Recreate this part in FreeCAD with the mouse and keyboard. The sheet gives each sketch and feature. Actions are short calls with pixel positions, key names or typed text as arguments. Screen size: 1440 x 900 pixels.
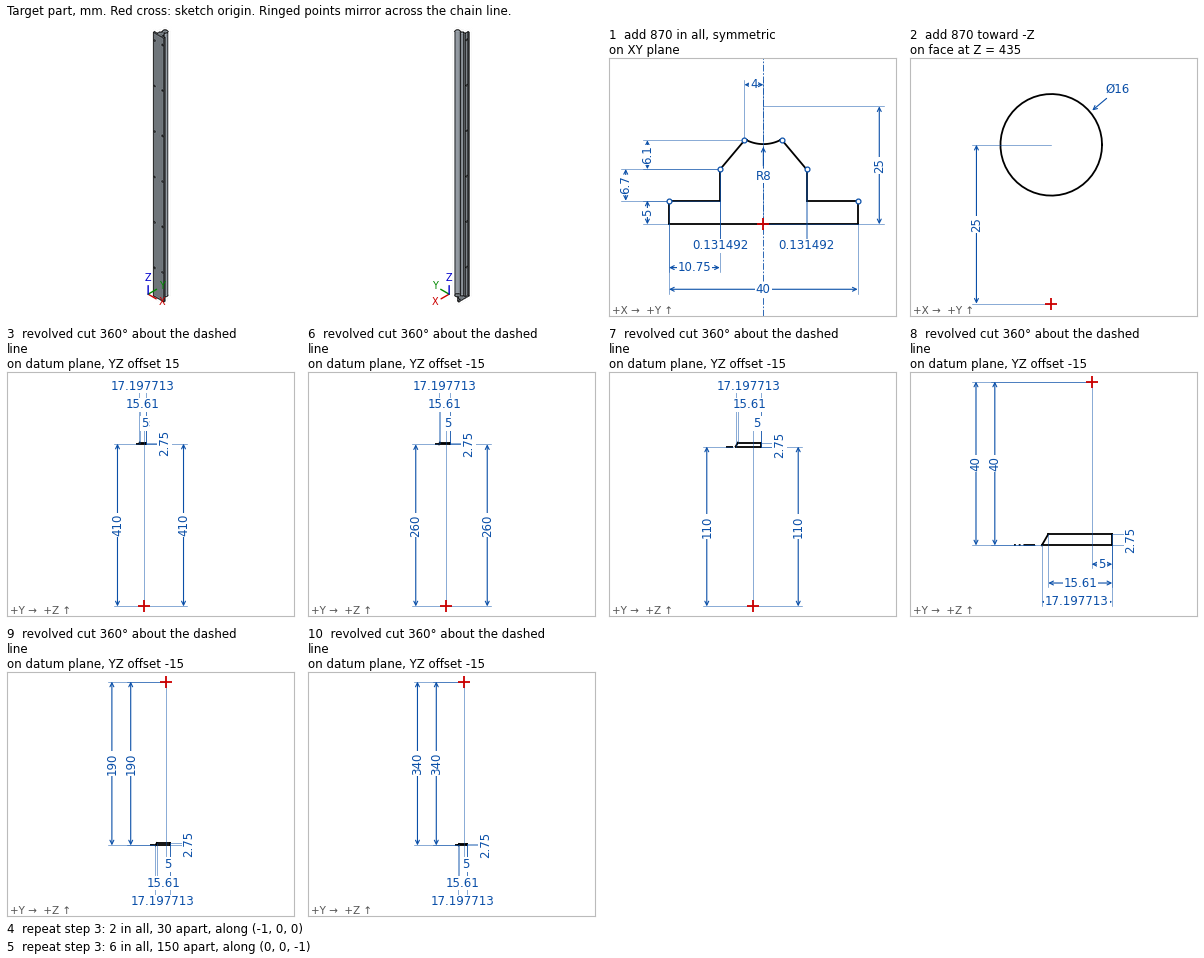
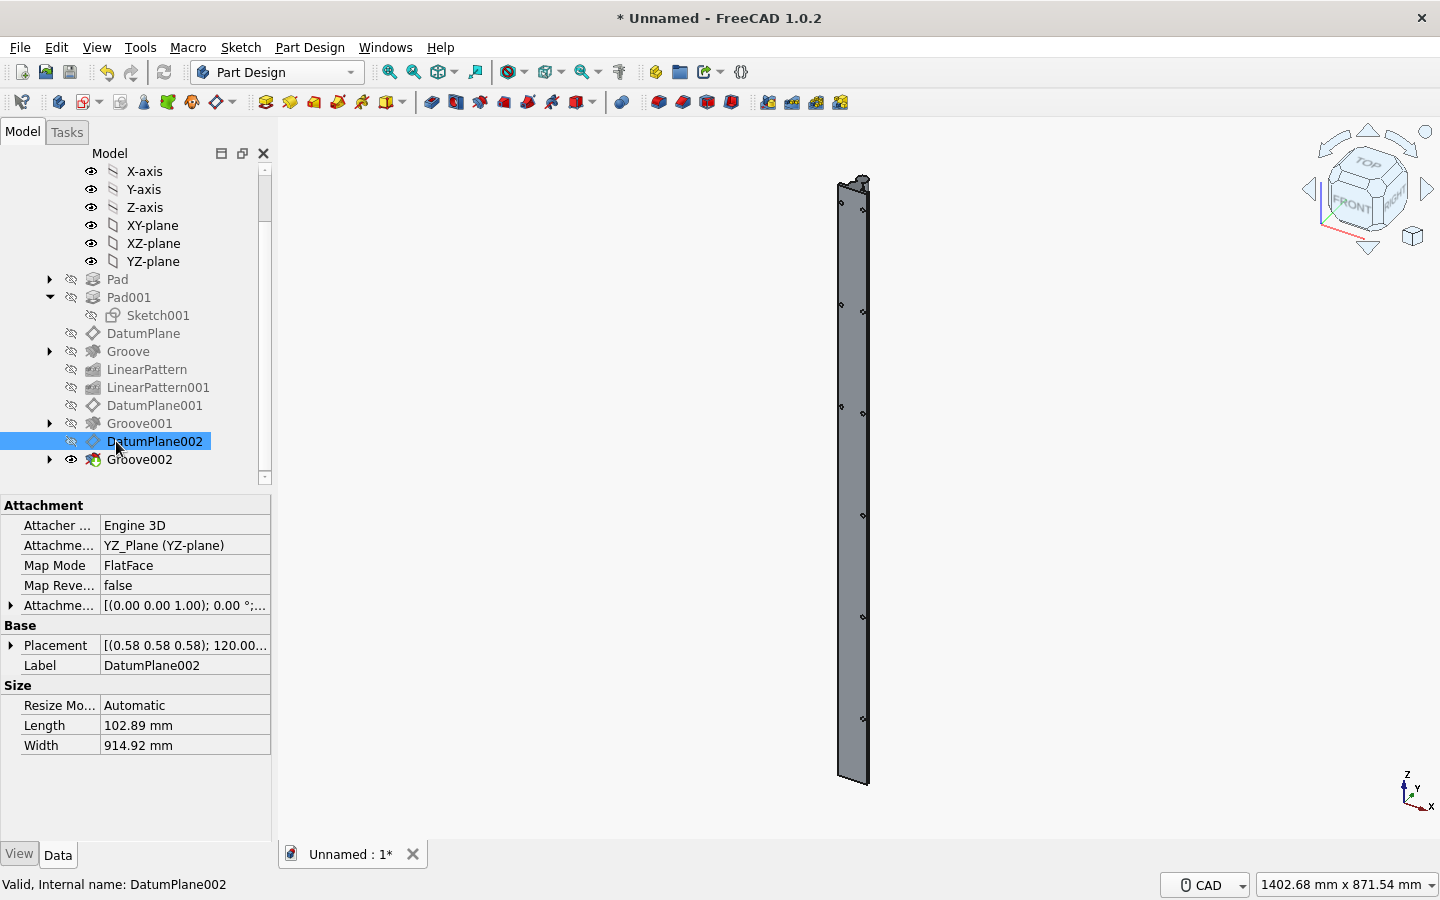
scroll(160, 311, down, 3)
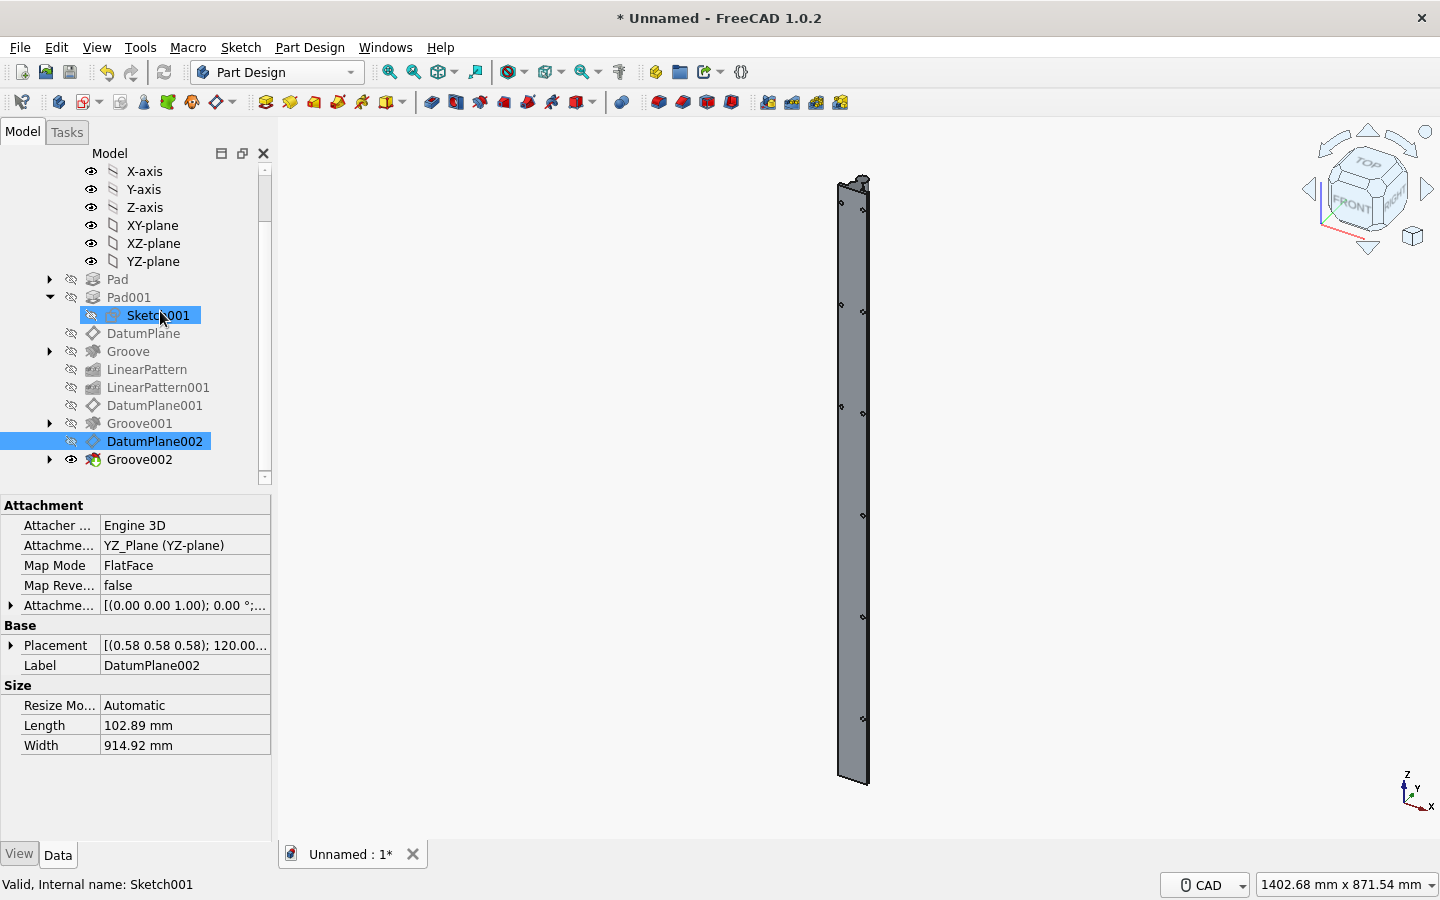
scroll(160, 311, up, 15)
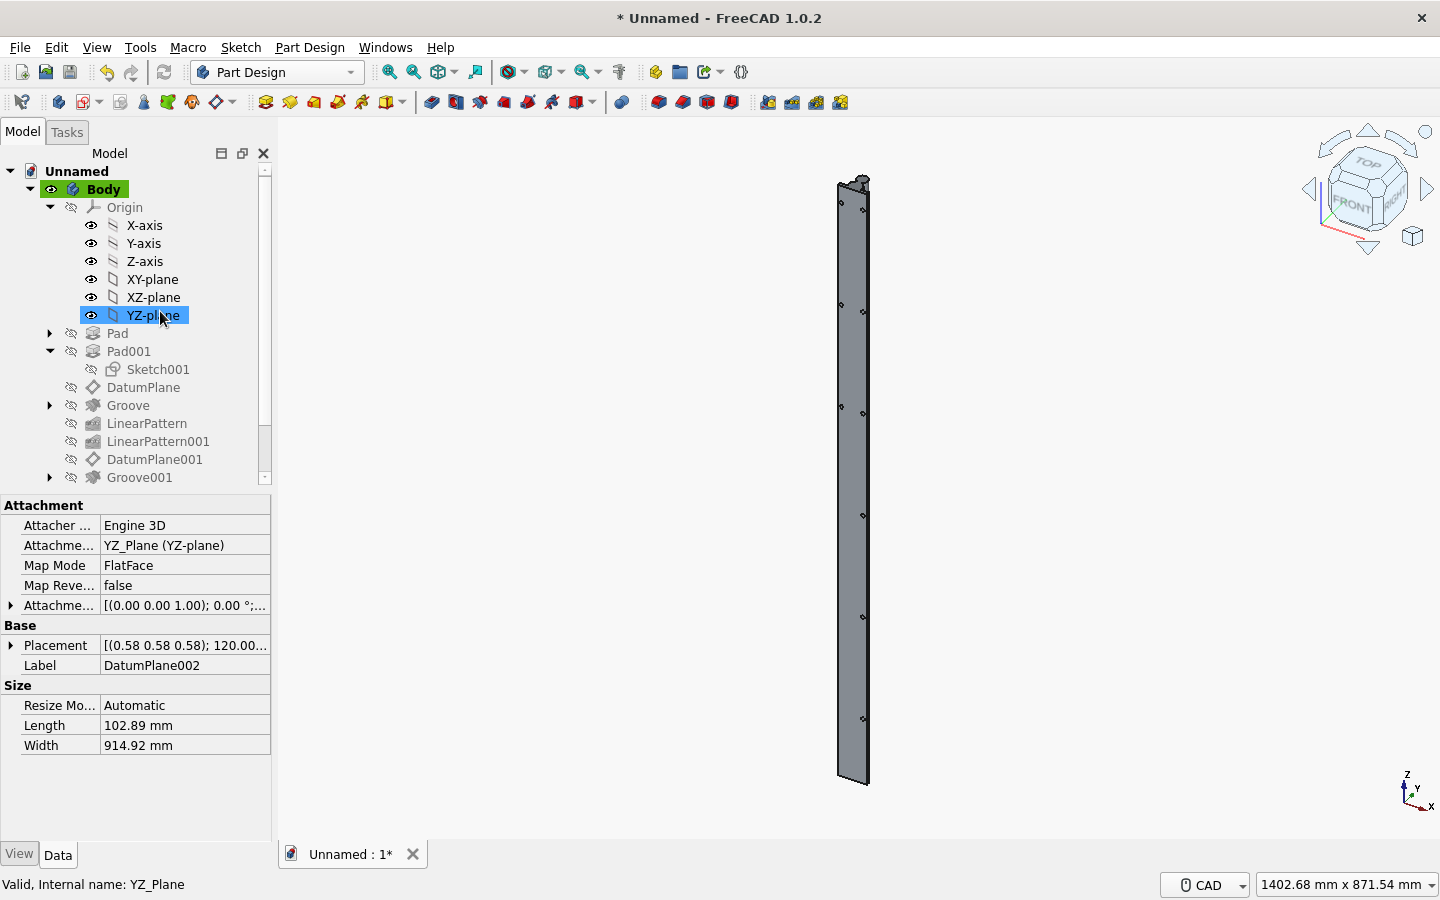
click(136, 315)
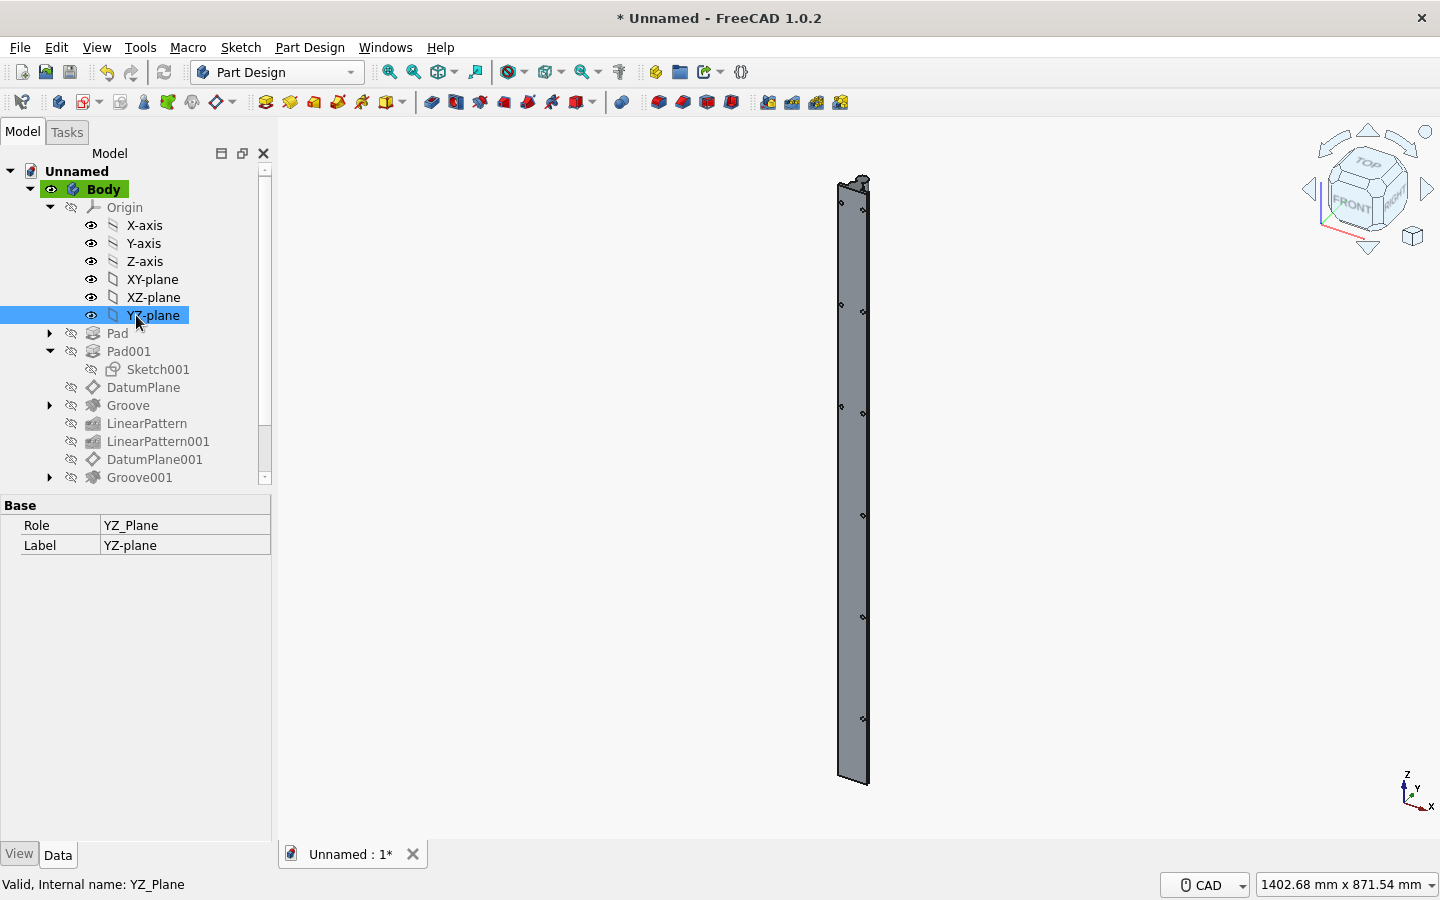
click(216, 102)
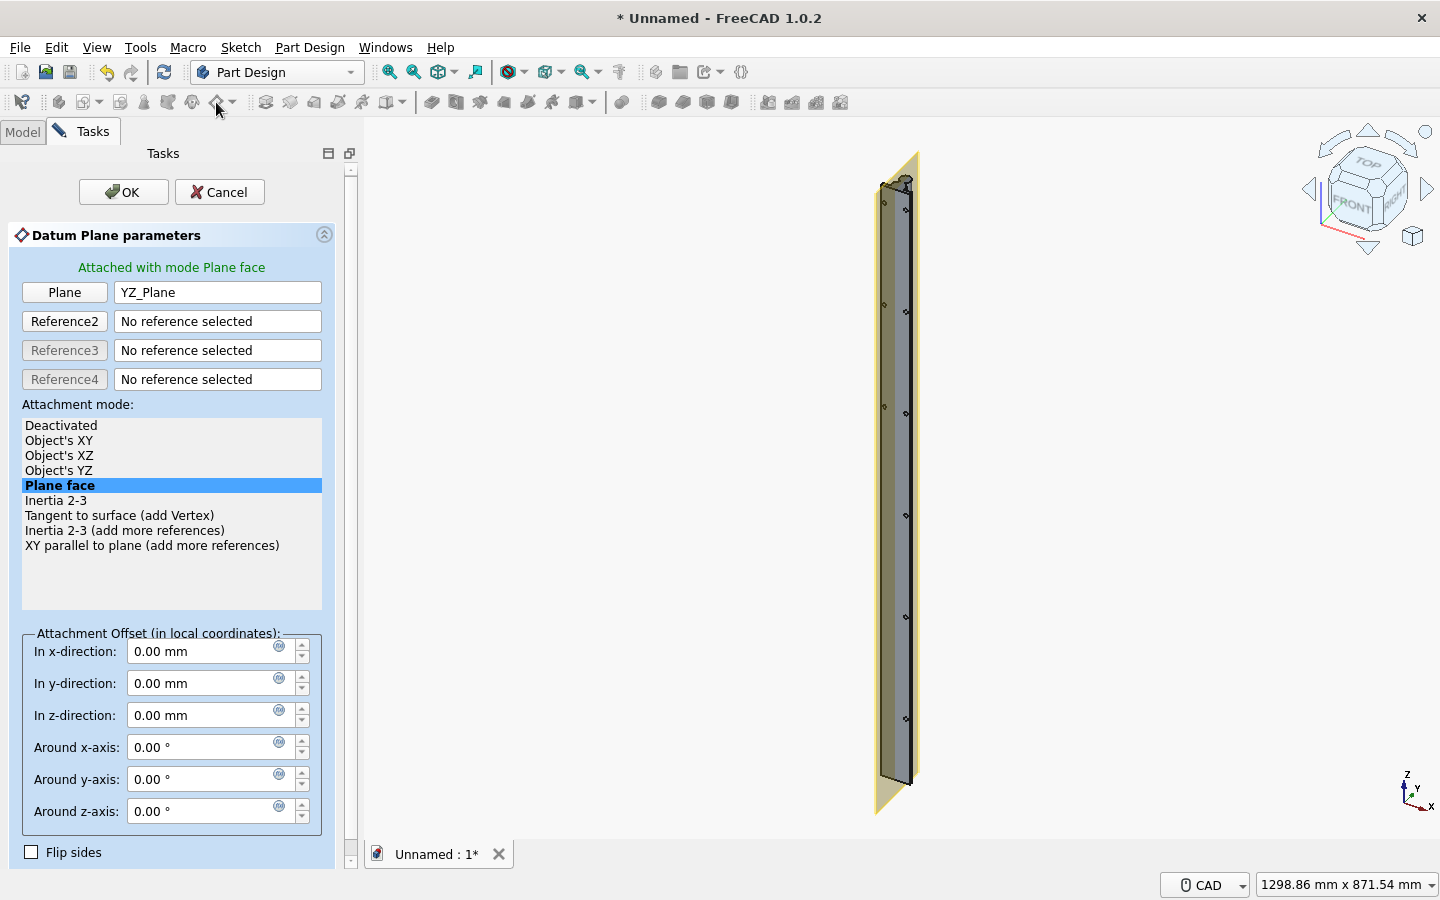
triple_click(210, 715)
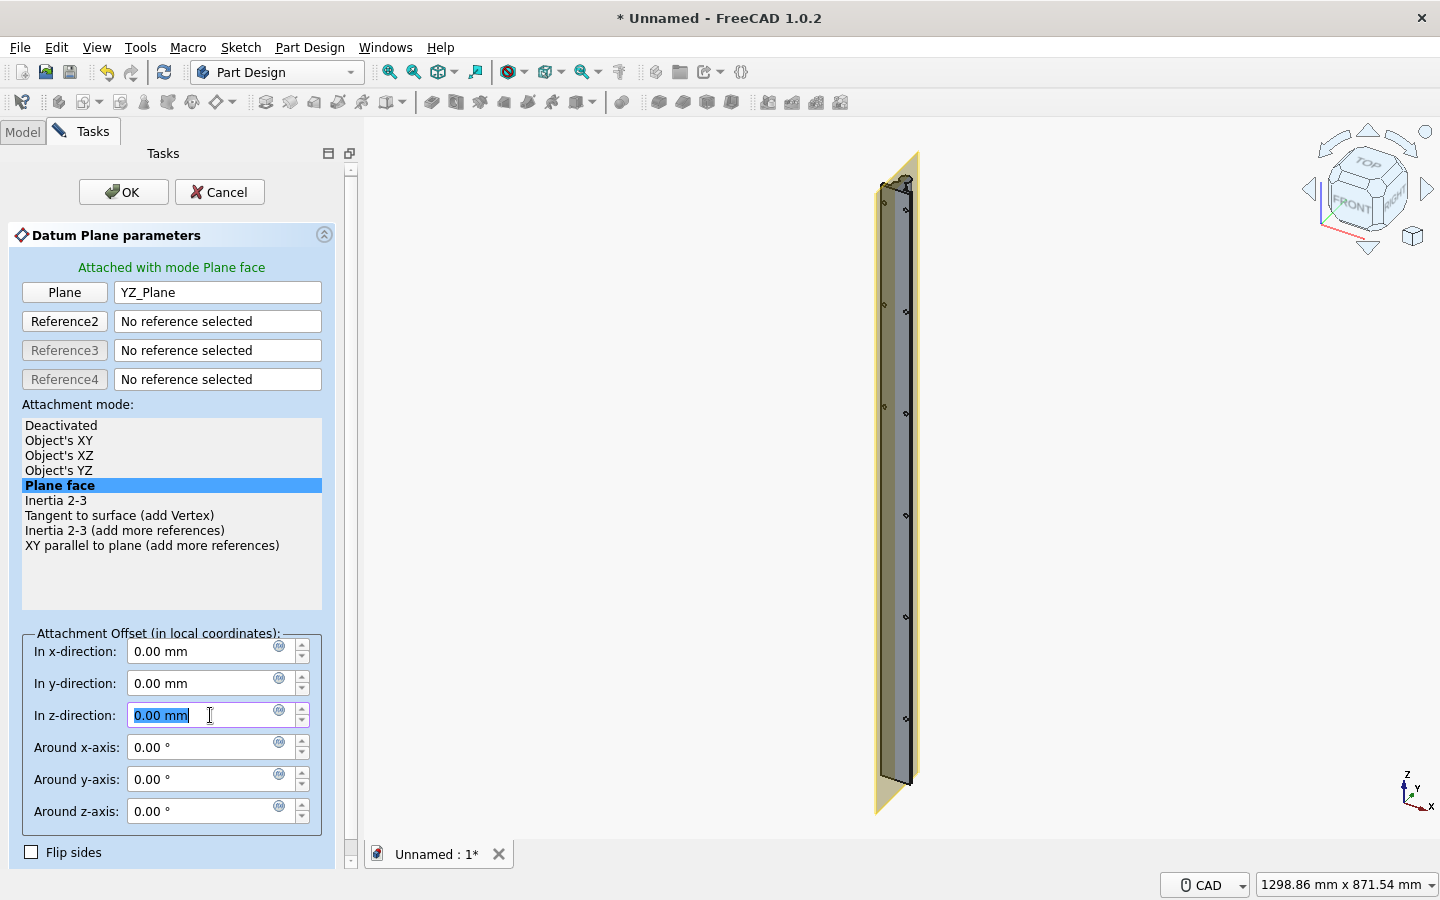
text(-15)
key(Tab)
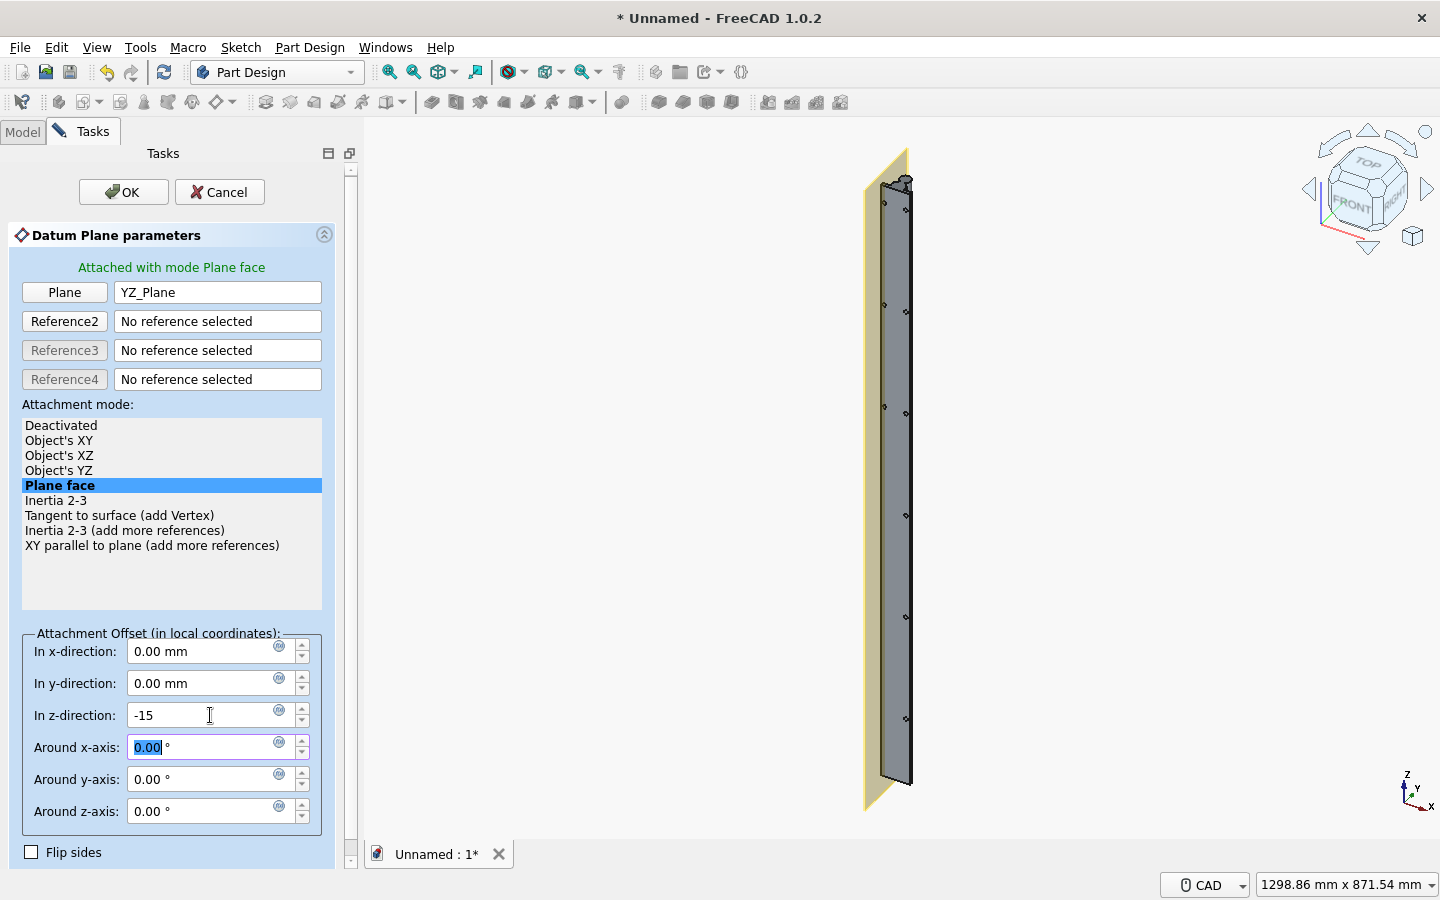
click(124, 192)